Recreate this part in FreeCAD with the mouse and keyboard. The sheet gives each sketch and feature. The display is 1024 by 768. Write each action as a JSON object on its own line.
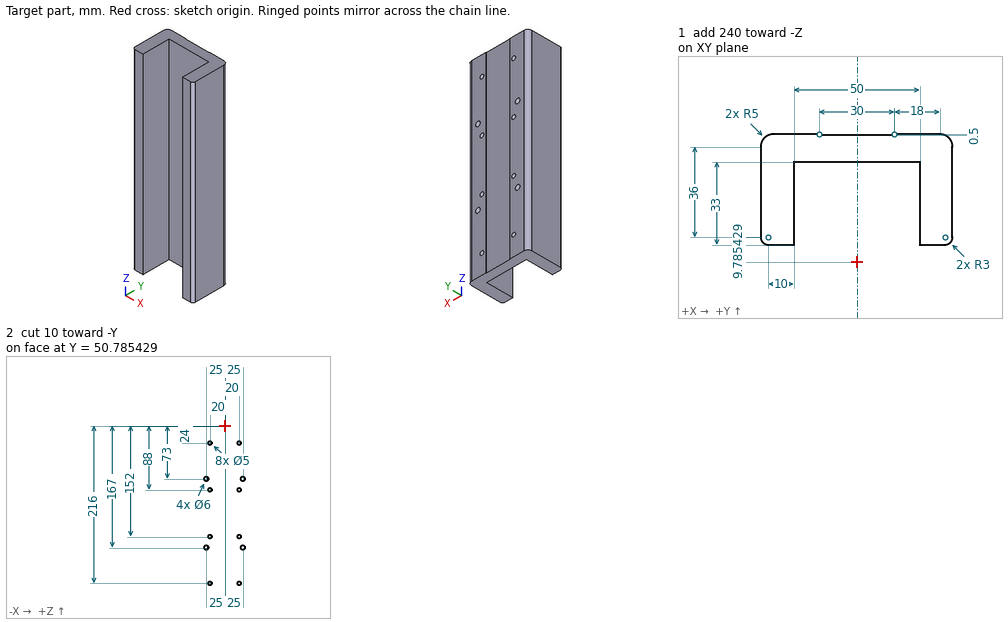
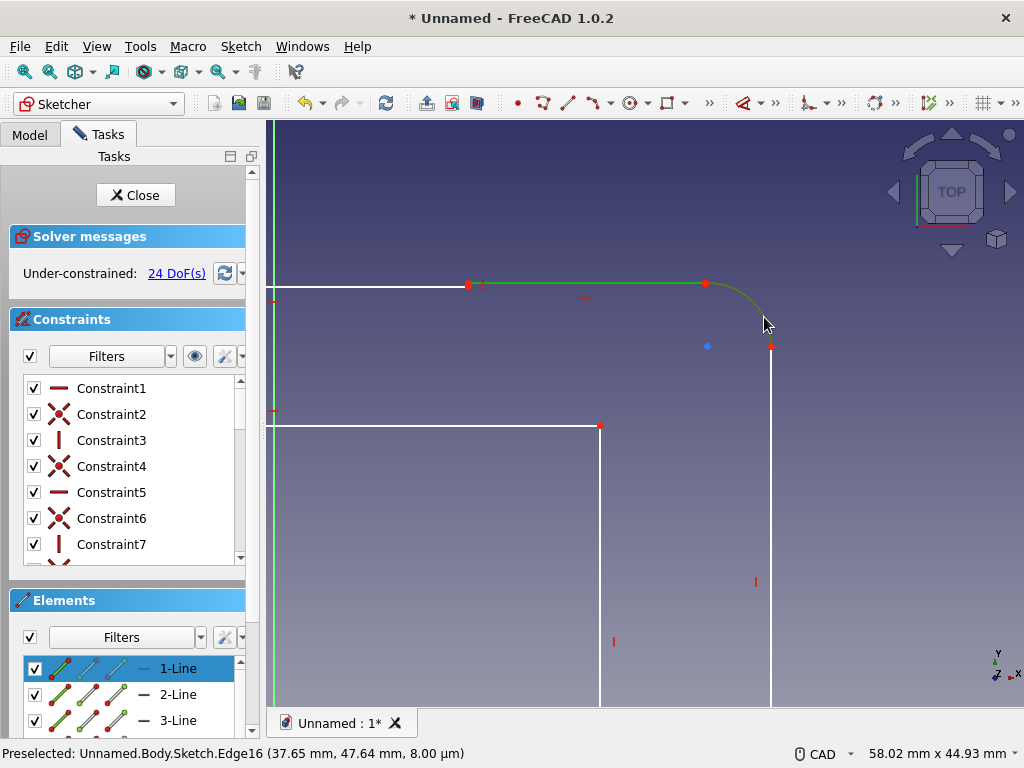
{"action": "key", "text": "t"}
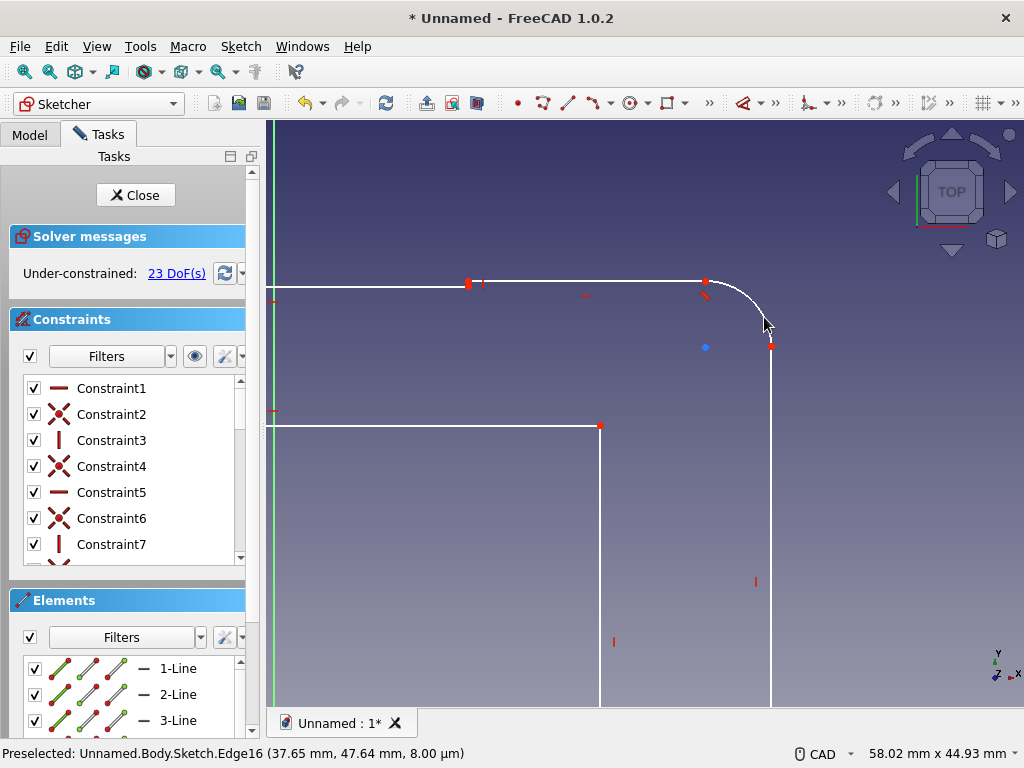
{"action": "scroll", "coordinate": [753, 298], "scroll_direction": "down", "scroll_amount": 5}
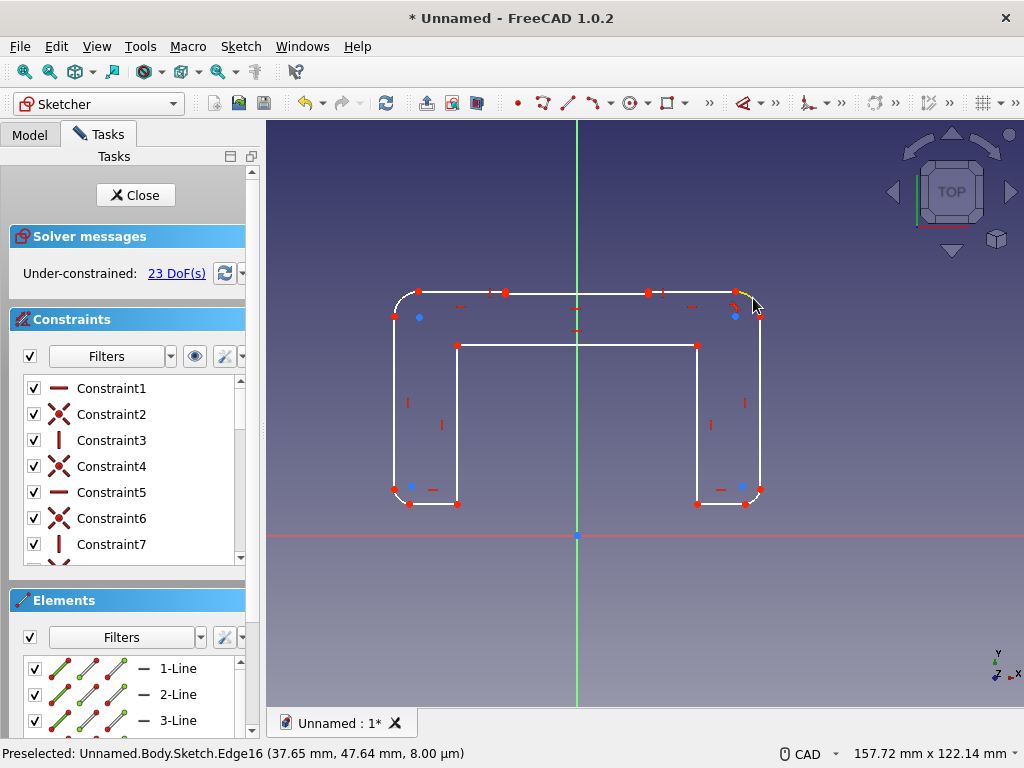
{"action": "left_click", "coordinate": [479, 292]}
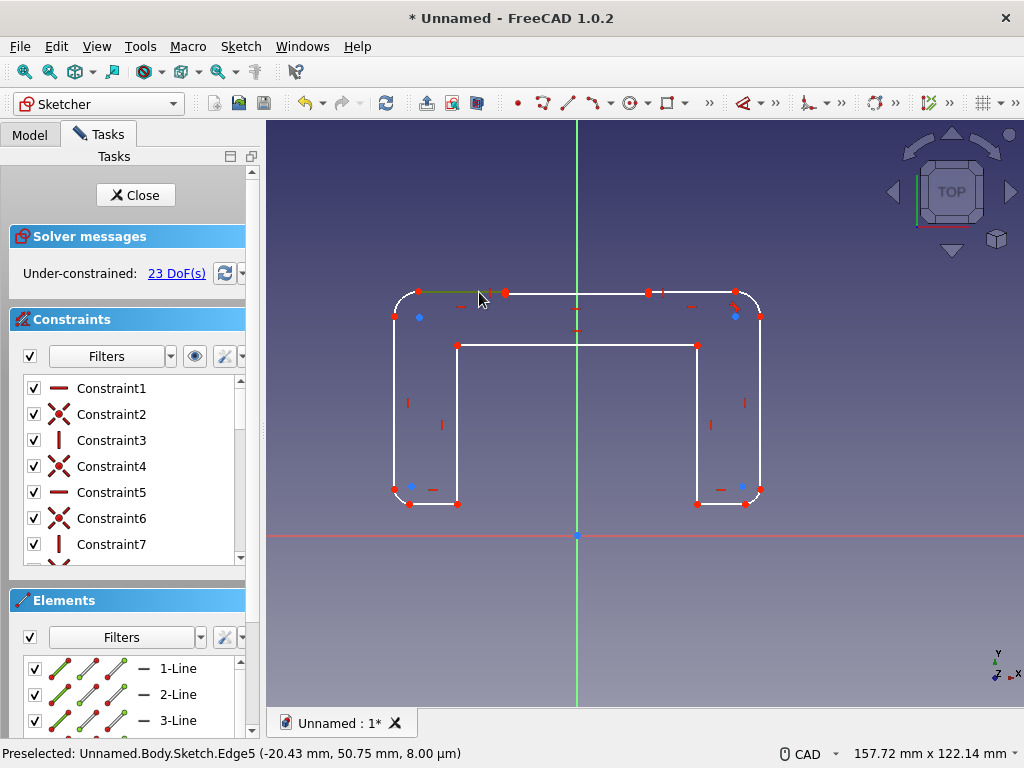
{"action": "scroll", "coordinate": [407, 295], "scroll_direction": "up", "scroll_amount": 2}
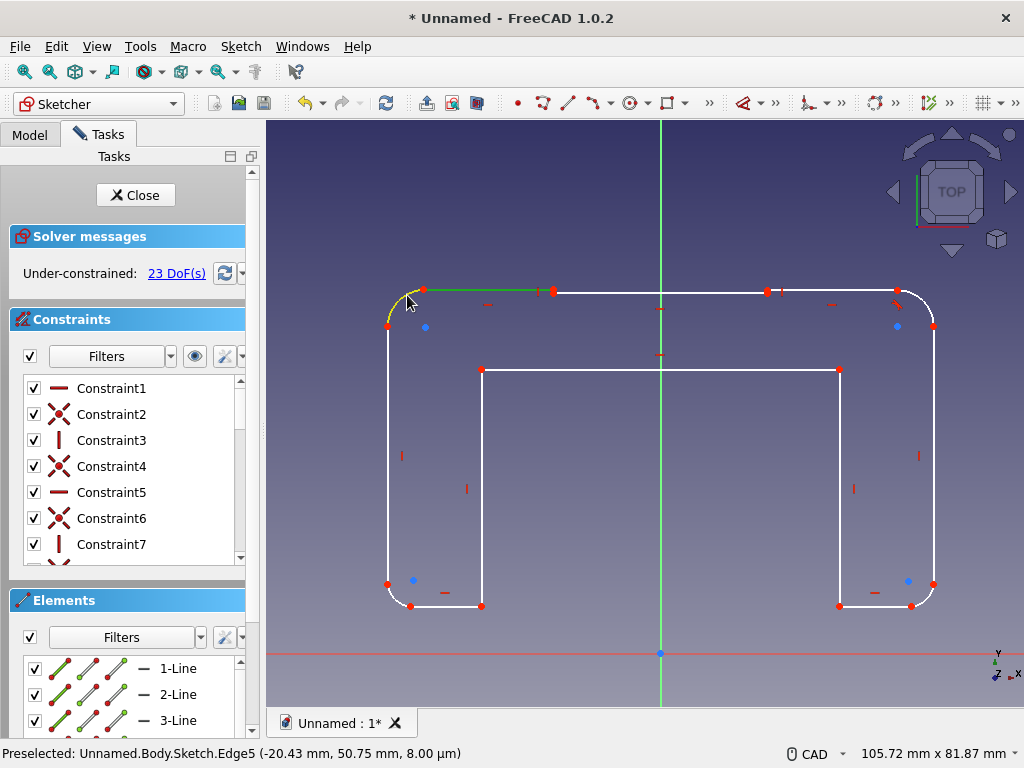
{"action": "left_click", "coordinate": [407, 294]}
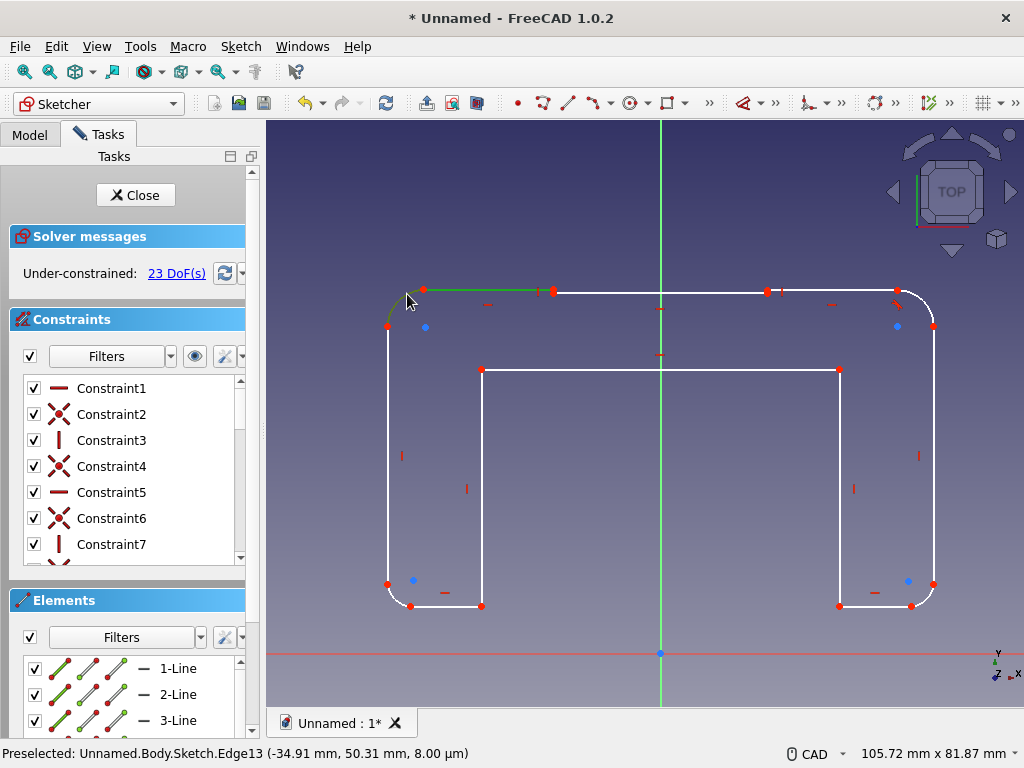
{"action": "key", "text": "t"}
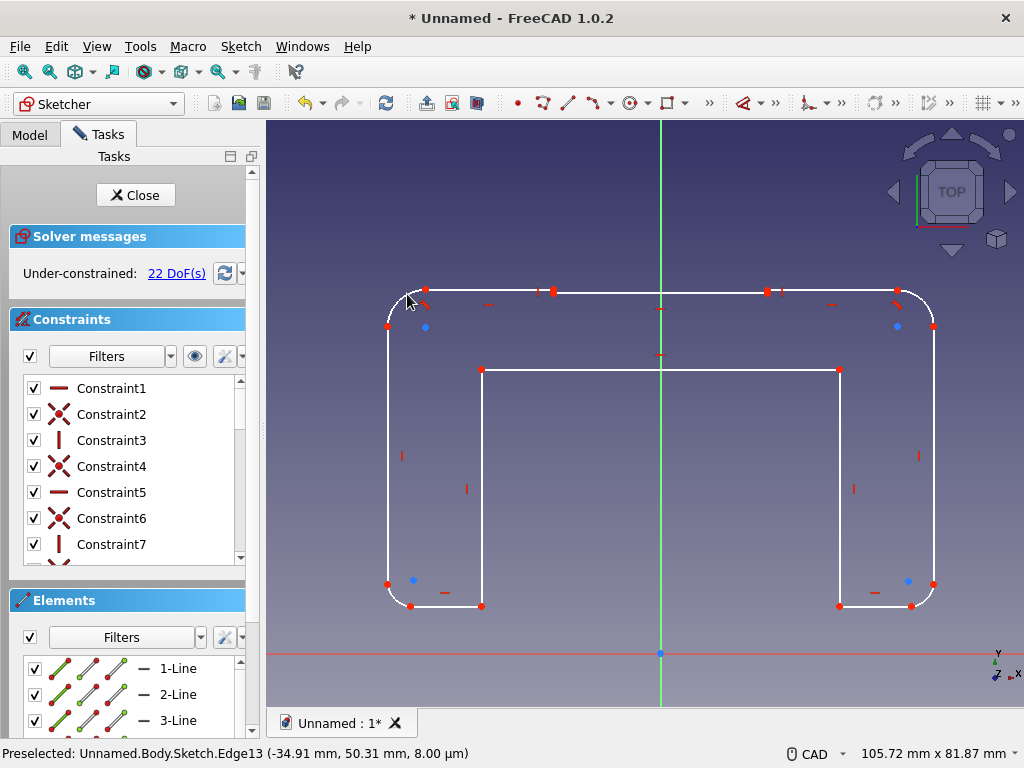
{"action": "left_click", "coordinate": [388, 404]}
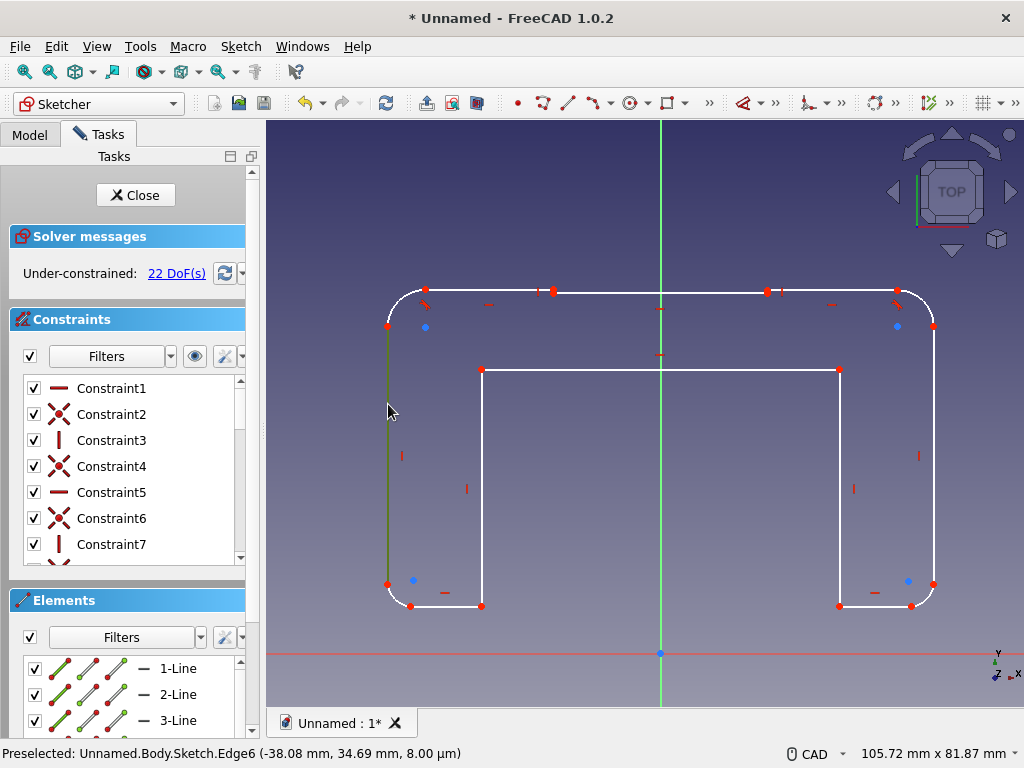
{"action": "left_click", "coordinate": [409, 294]}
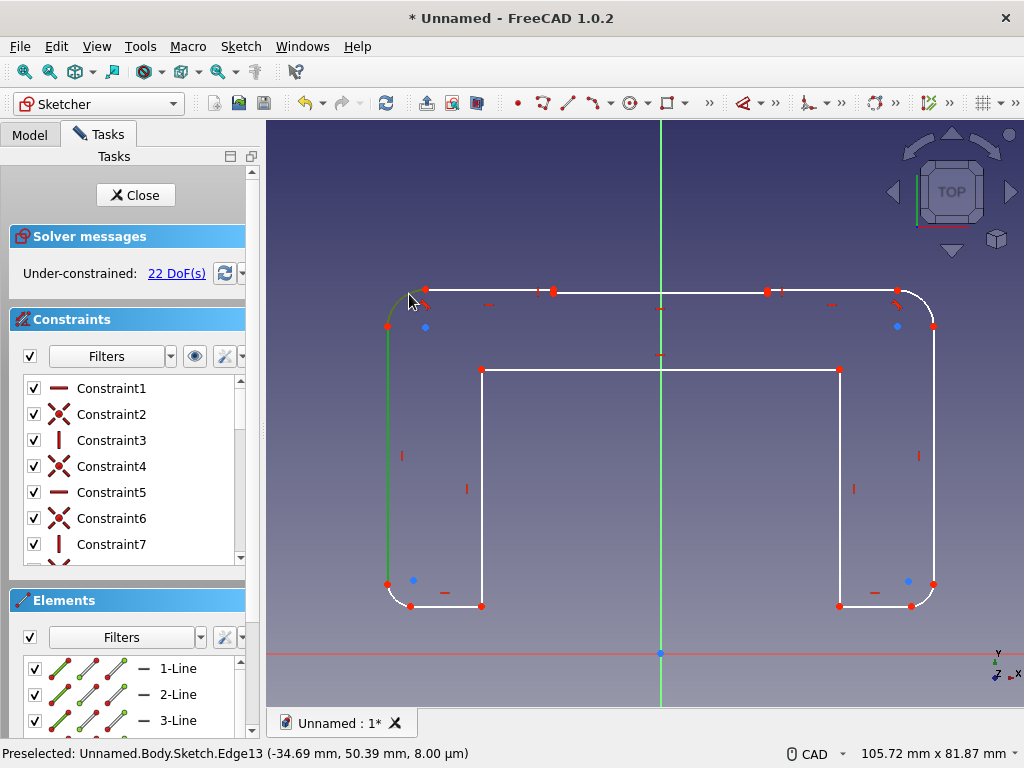
{"action": "key", "text": "t"}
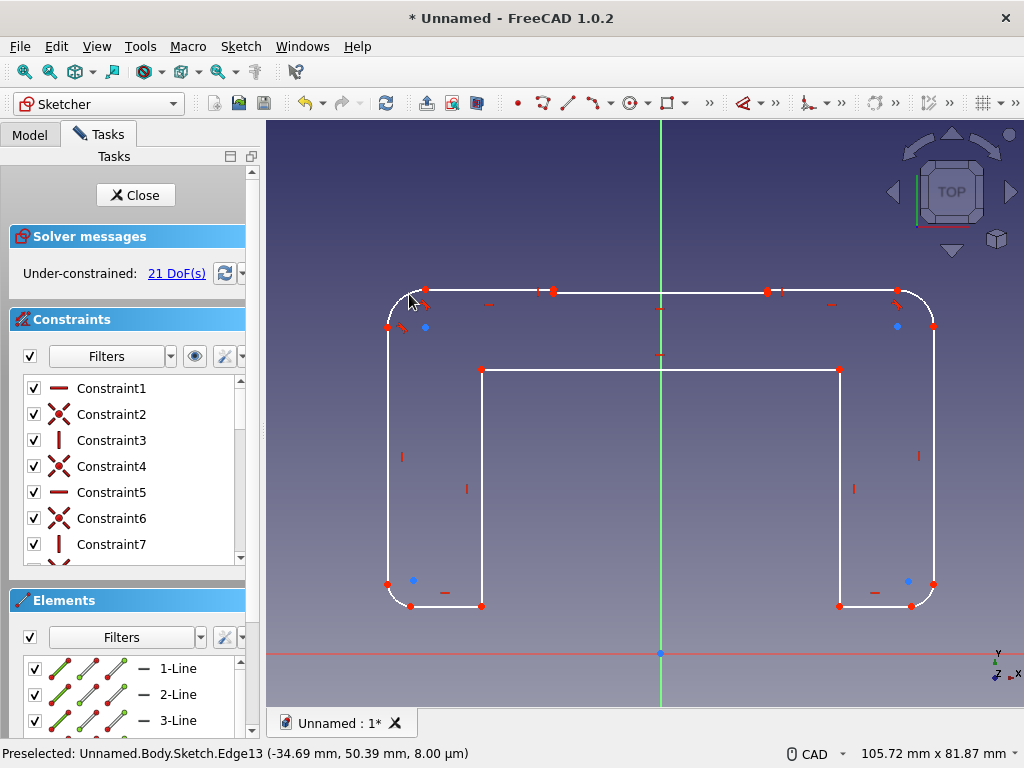
{"action": "left_click", "coordinate": [388, 405]}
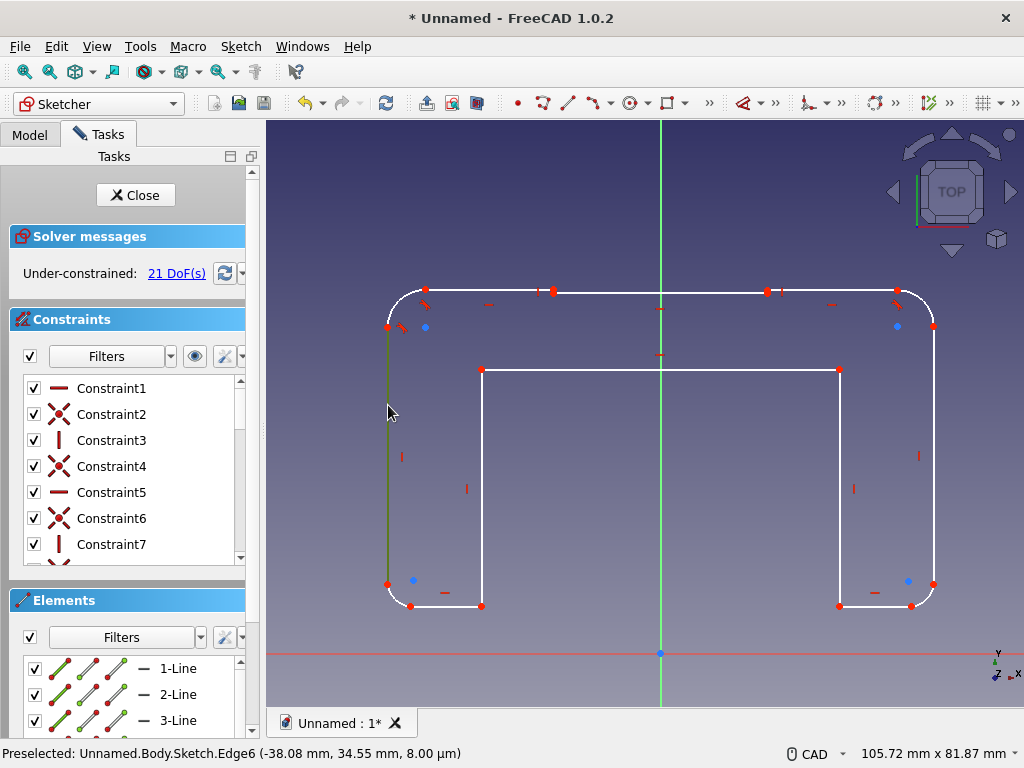
{"action": "scroll", "coordinate": [391, 594], "scroll_direction": "up", "scroll_amount": 2}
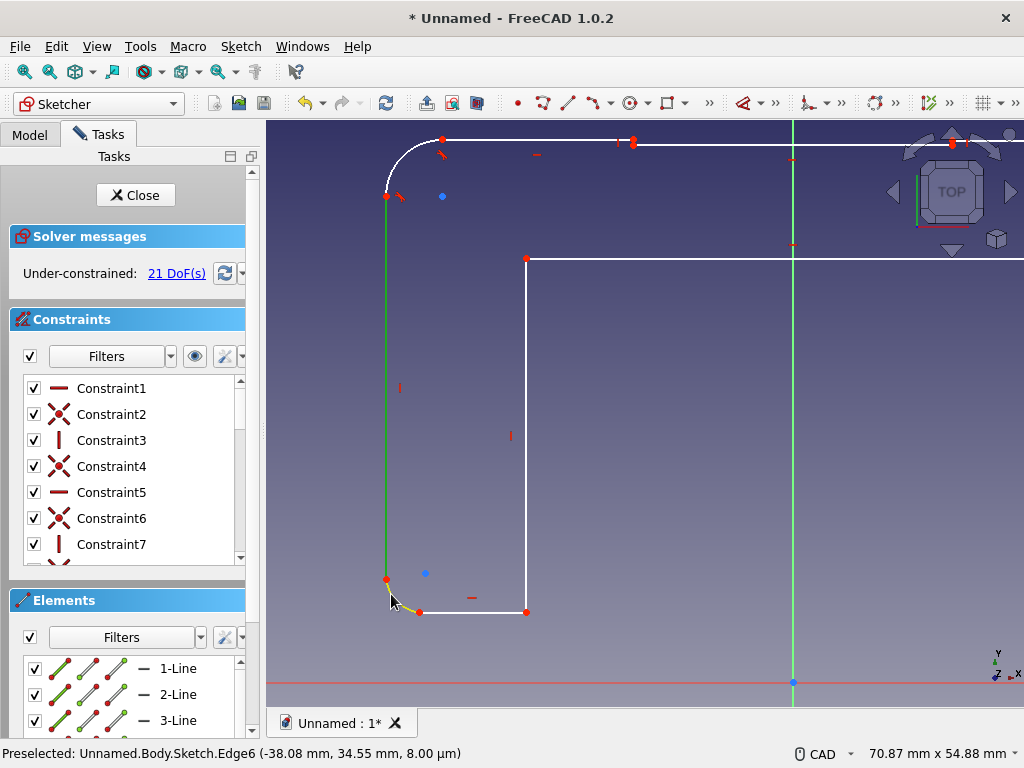
{"action": "left_click", "coordinate": [391, 594]}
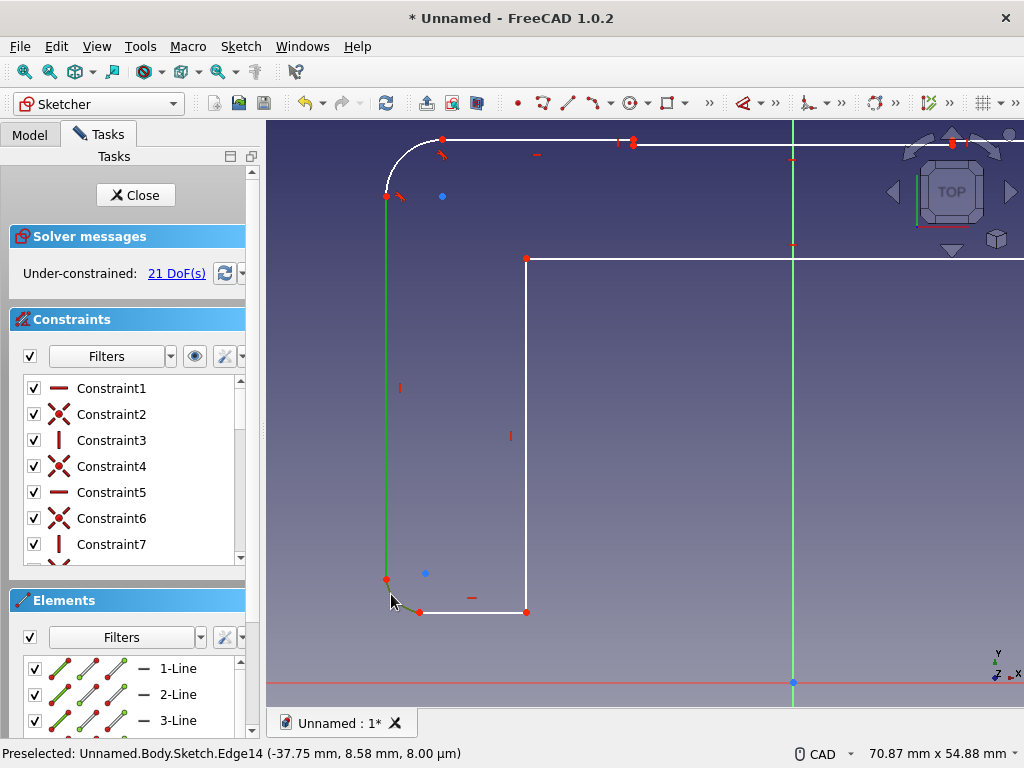
{"action": "key", "text": "t"}